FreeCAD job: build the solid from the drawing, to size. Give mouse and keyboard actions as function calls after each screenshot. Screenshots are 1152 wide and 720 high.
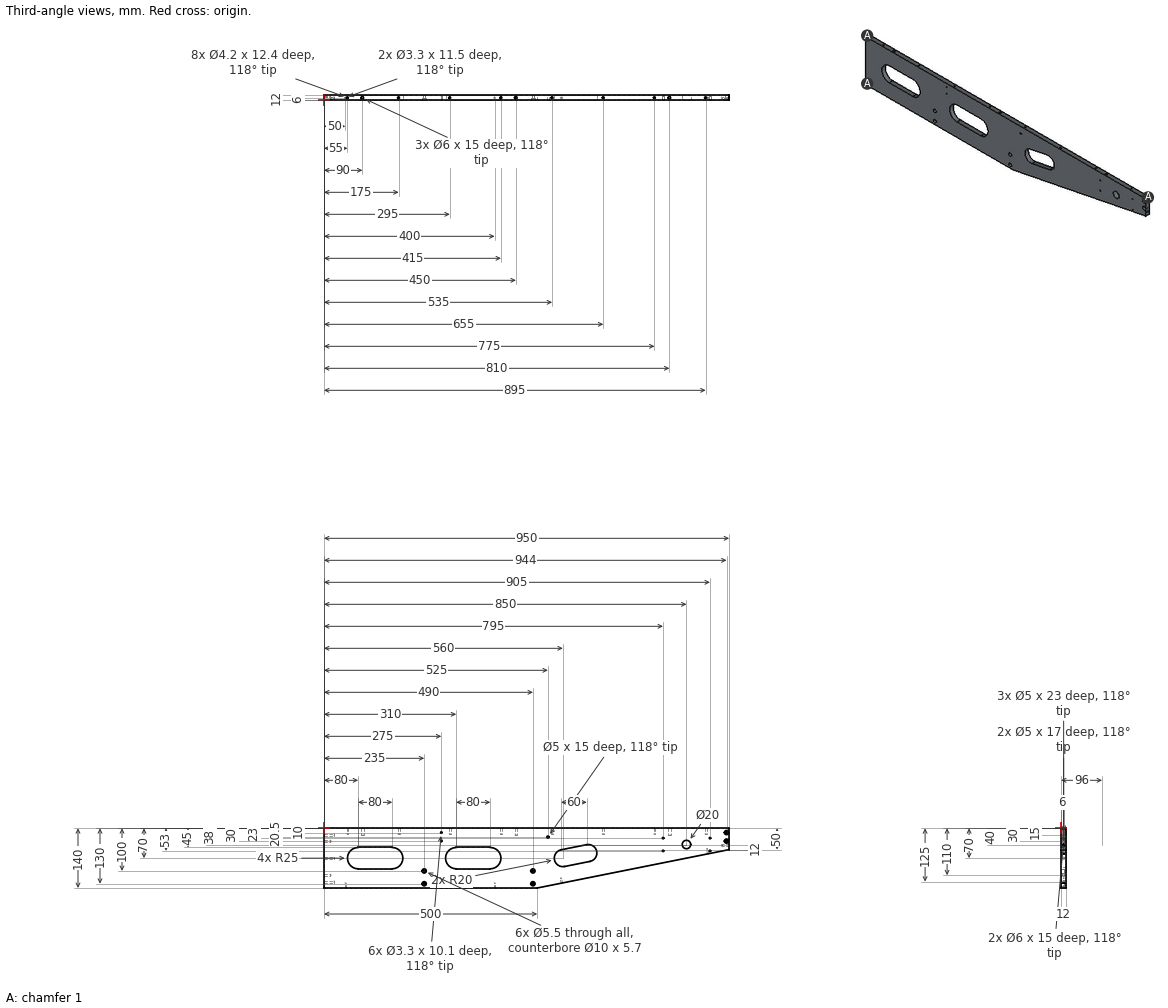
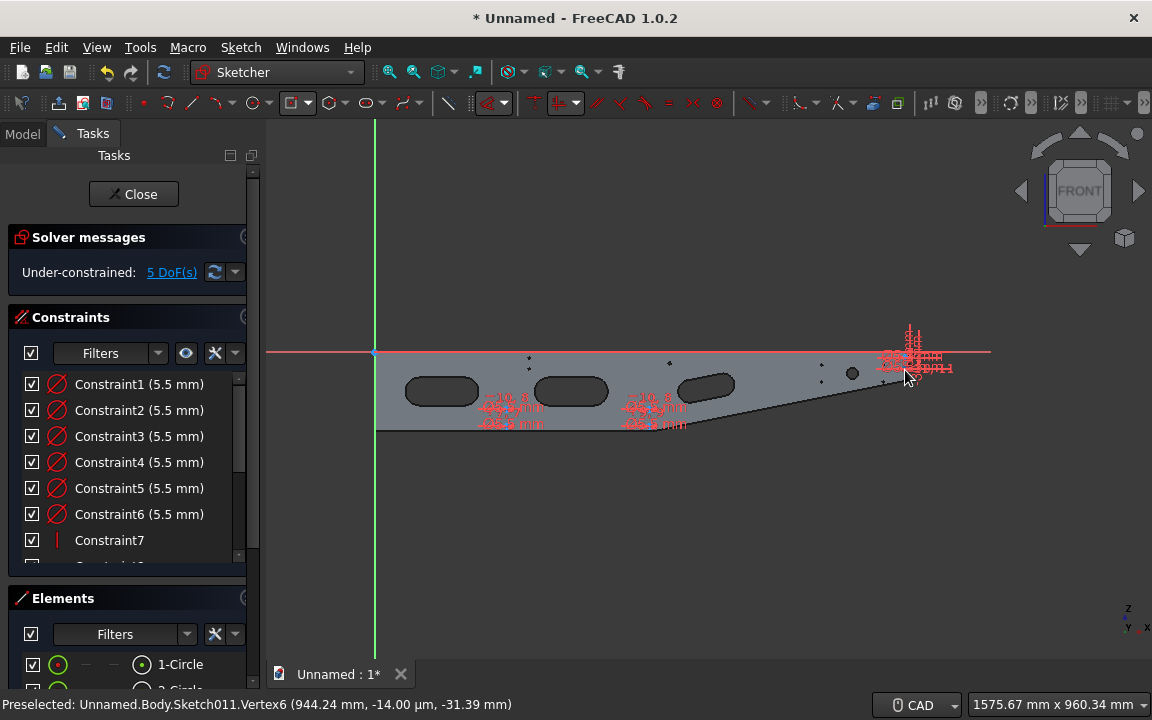
click(507, 409)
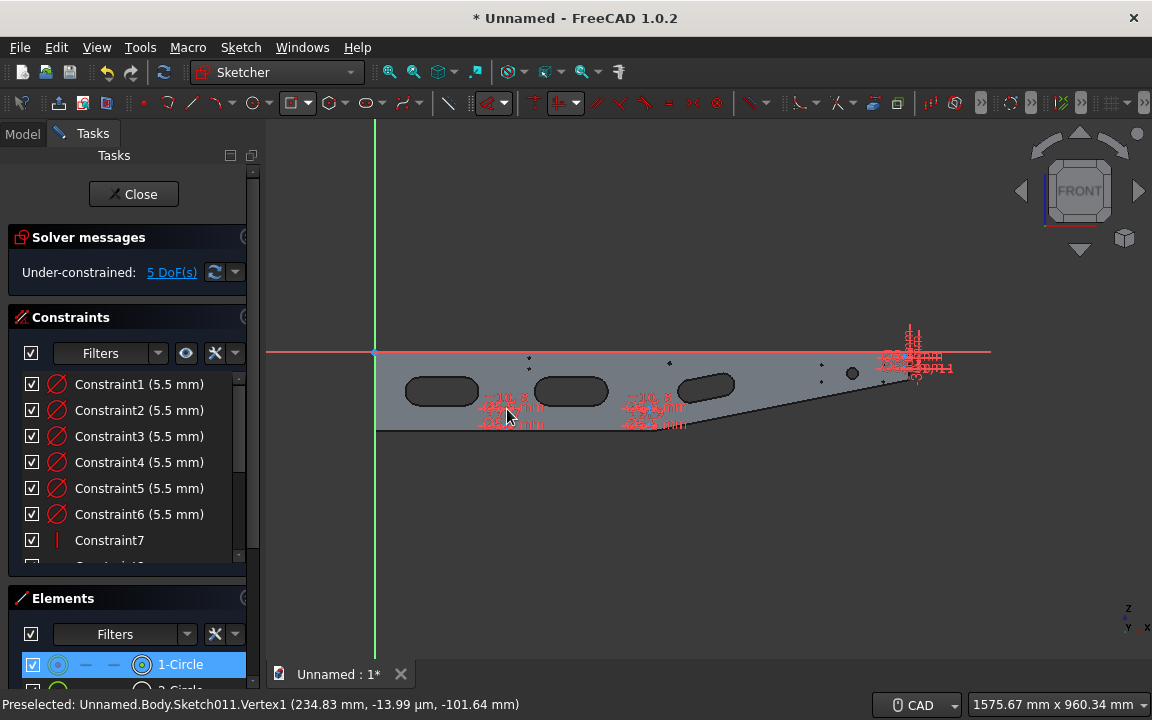
key(l)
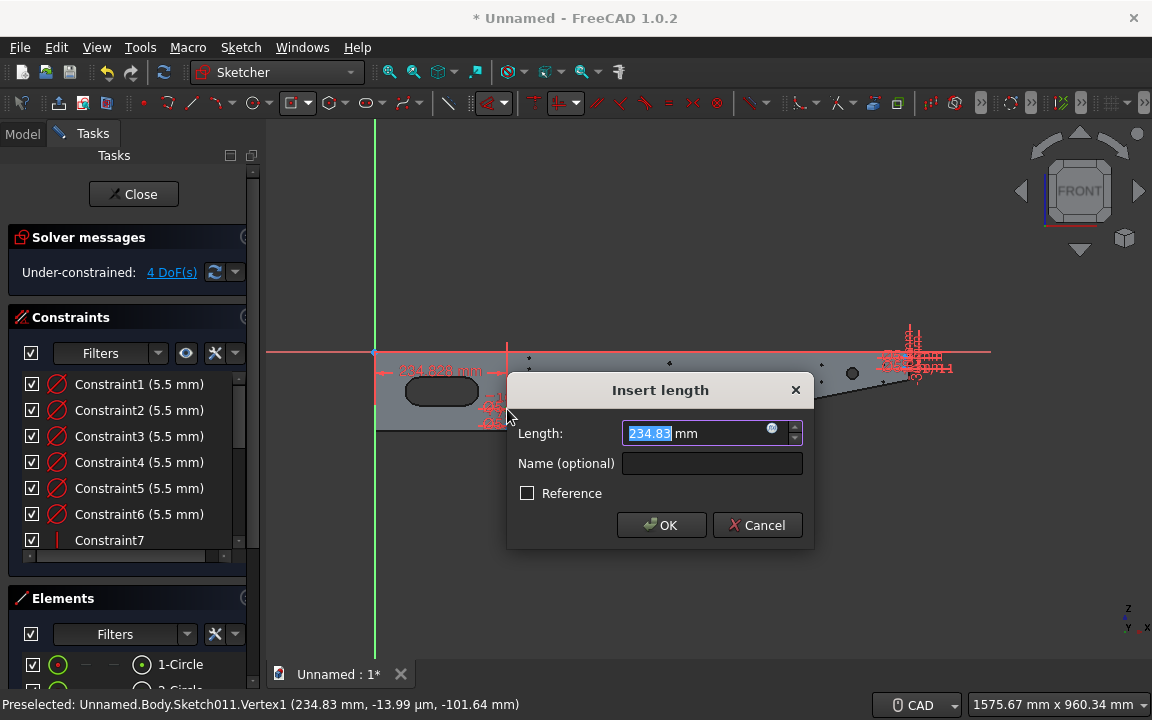
text(235)
key(Return)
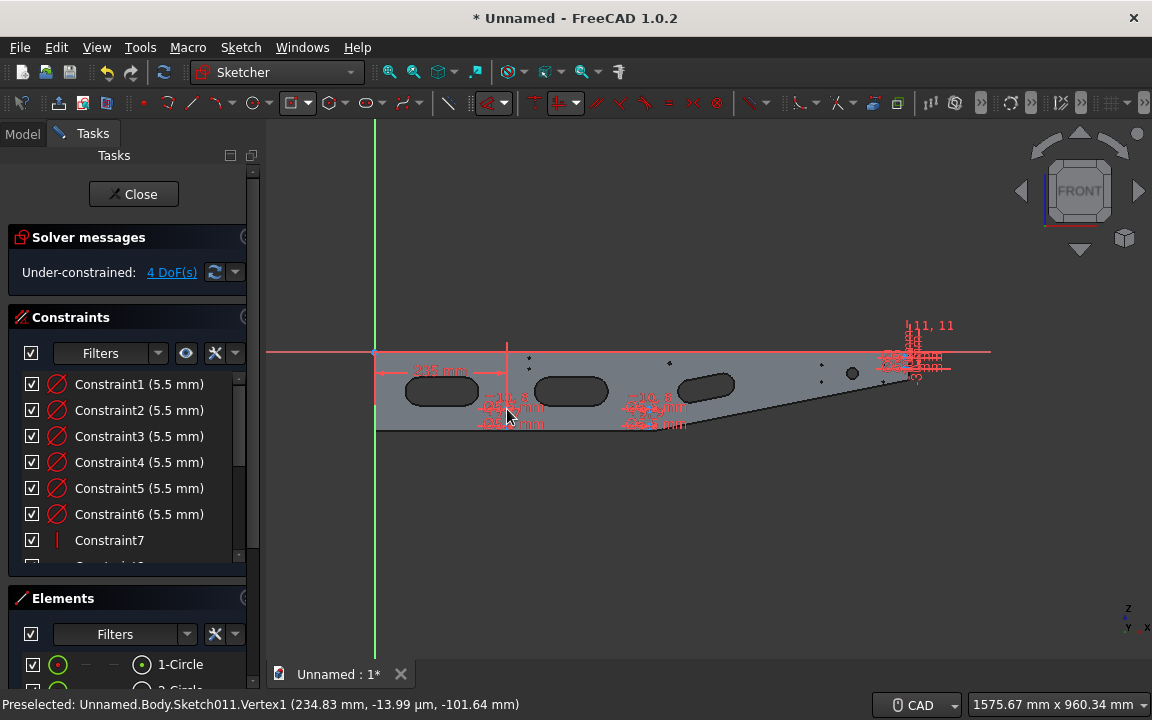
click(507, 409)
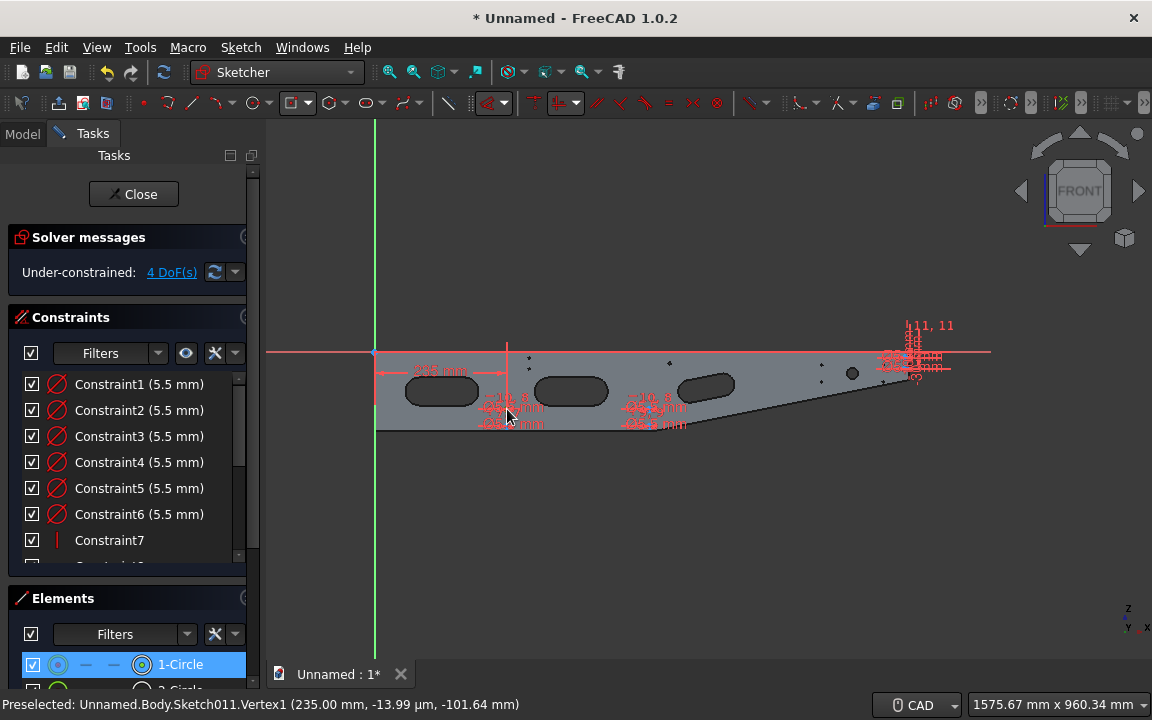
click(506, 104)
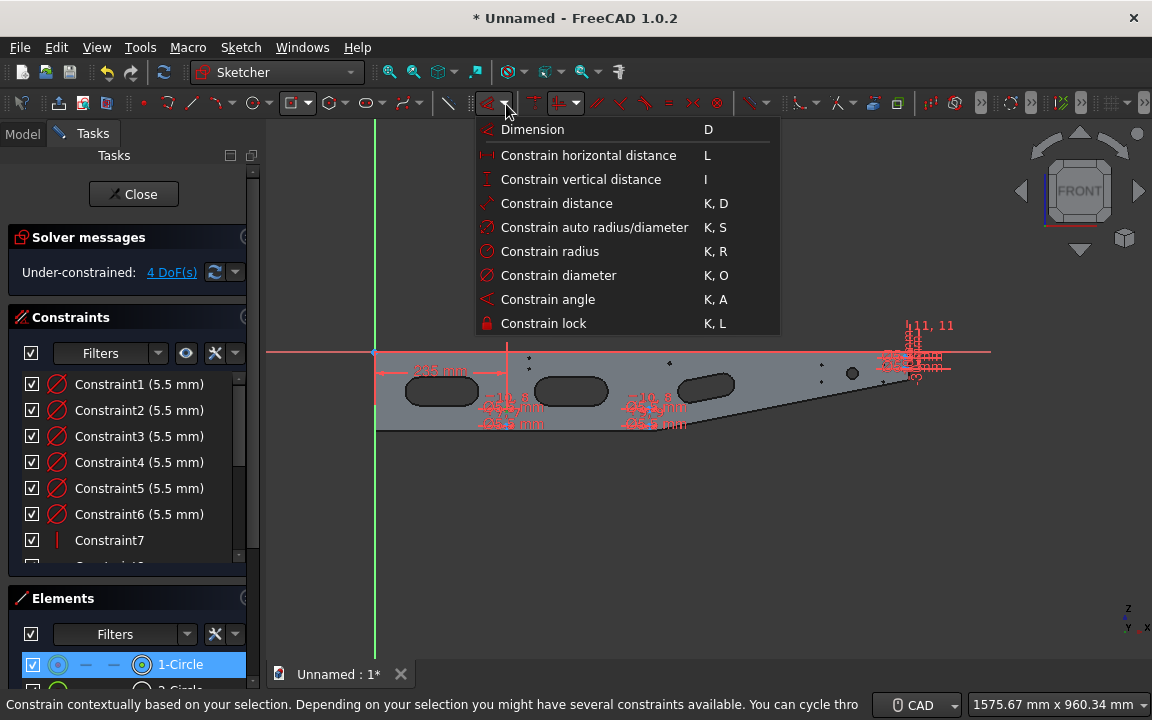
click(628, 179)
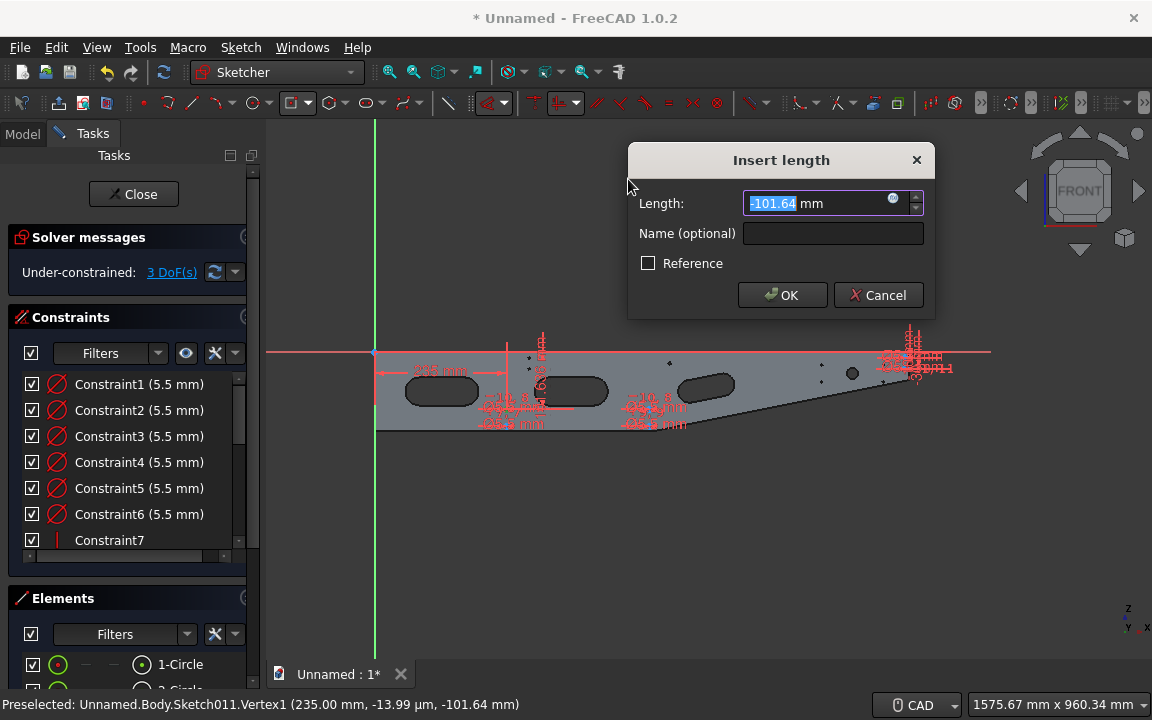
text(-100)
key(Return)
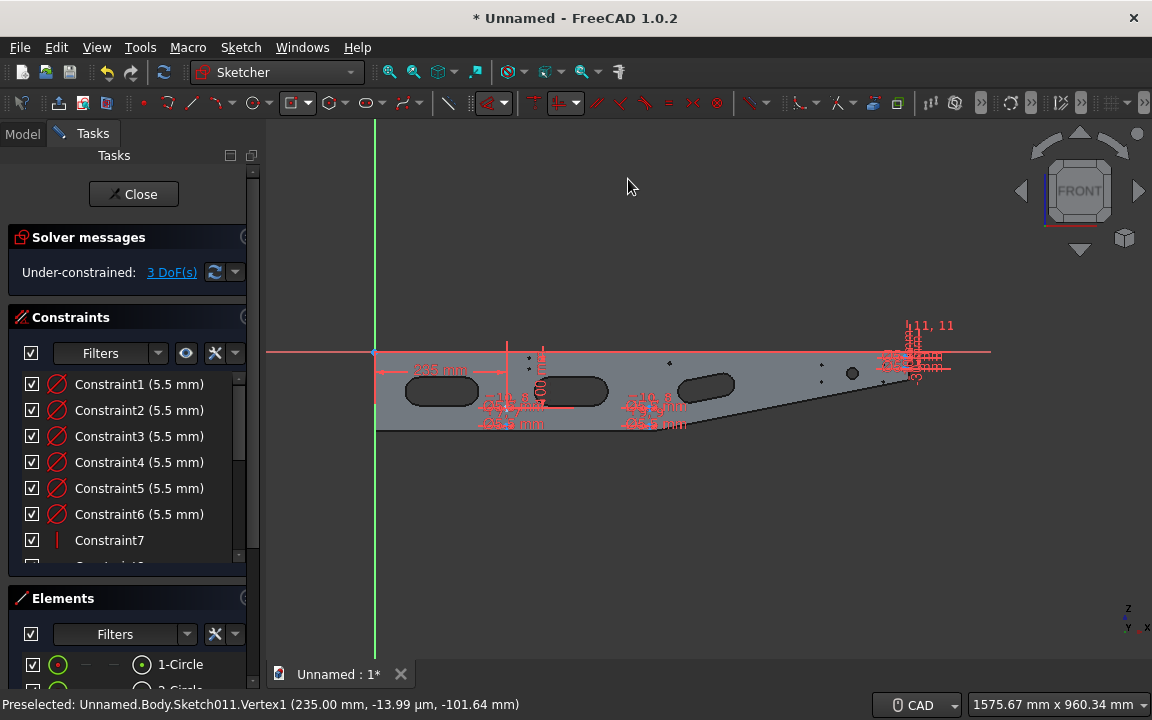
click(507, 426)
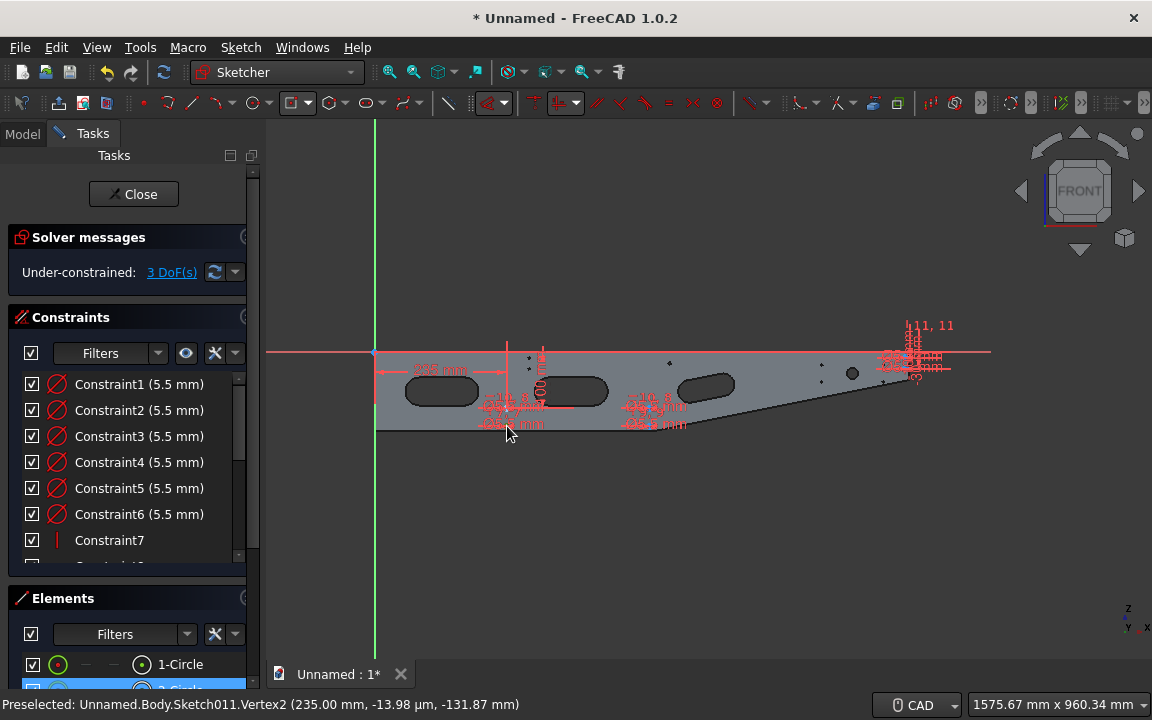
key(i)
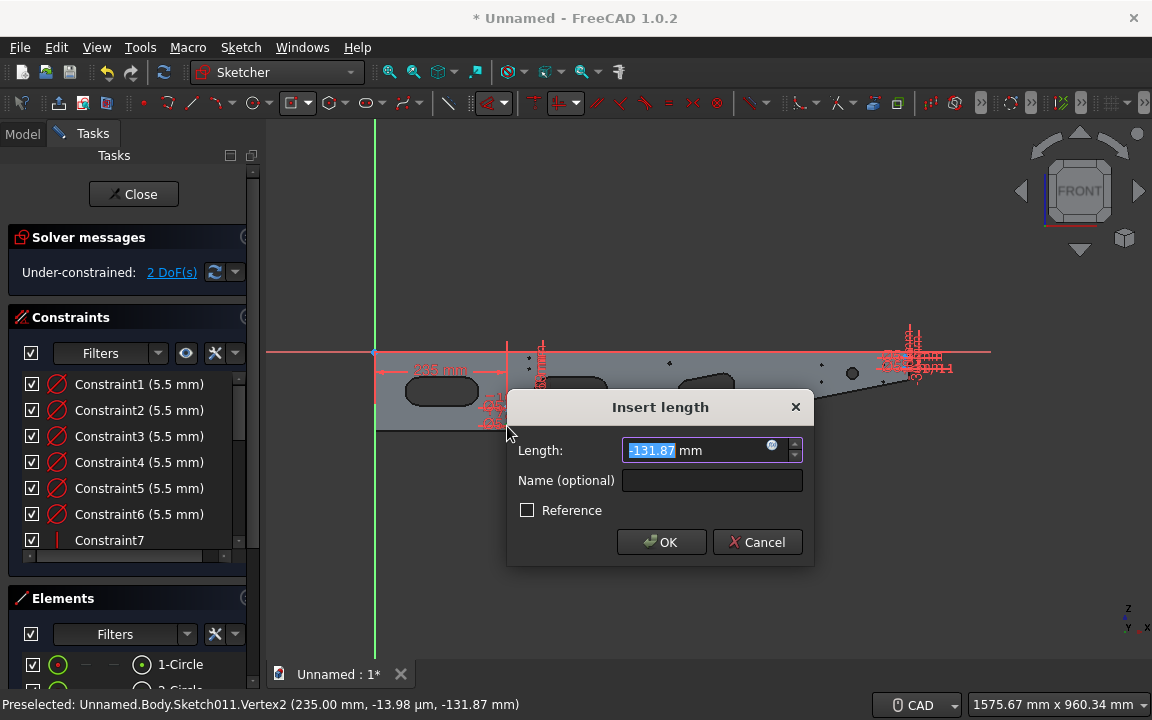
text(-130)
key(Return)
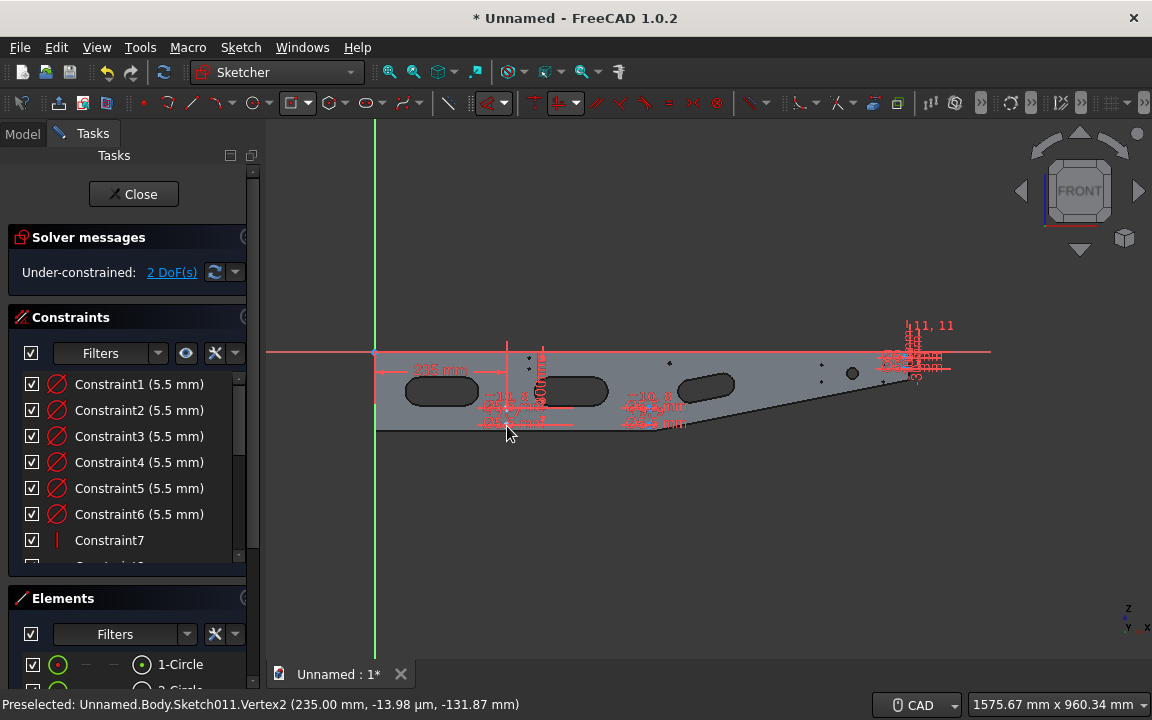
scroll(650, 408, up, 4)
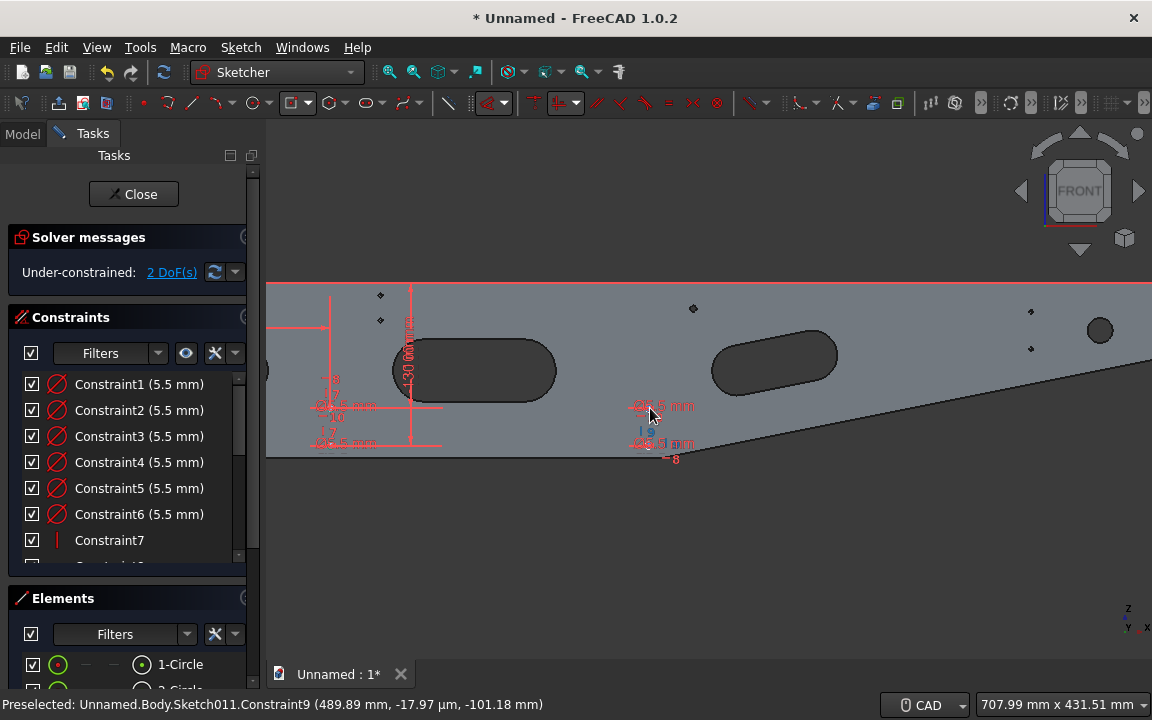
click(649, 408)